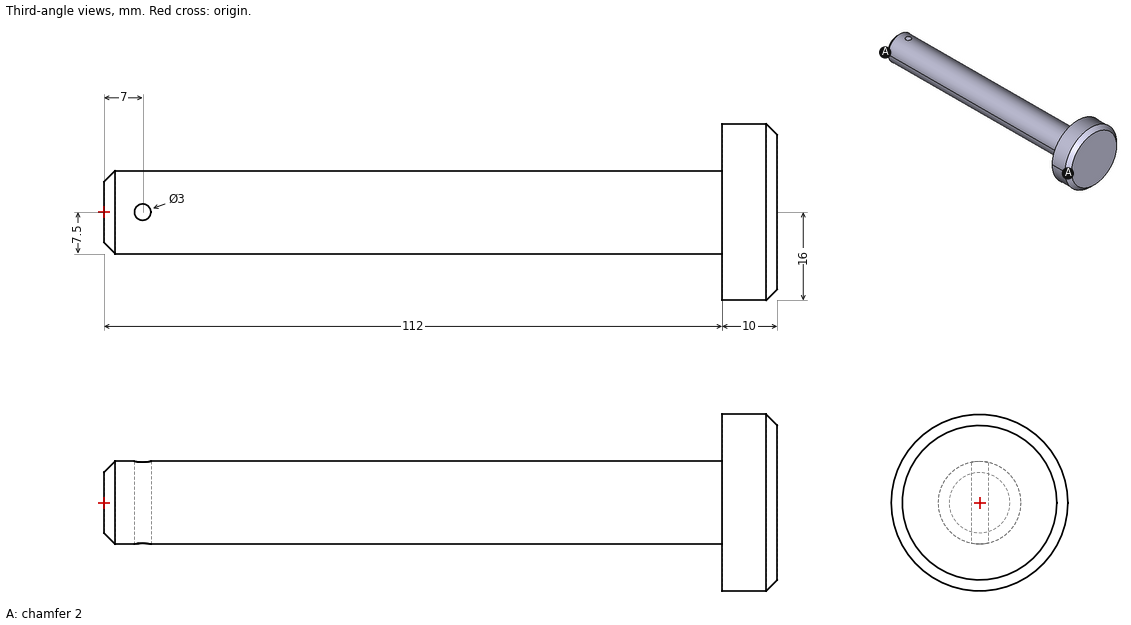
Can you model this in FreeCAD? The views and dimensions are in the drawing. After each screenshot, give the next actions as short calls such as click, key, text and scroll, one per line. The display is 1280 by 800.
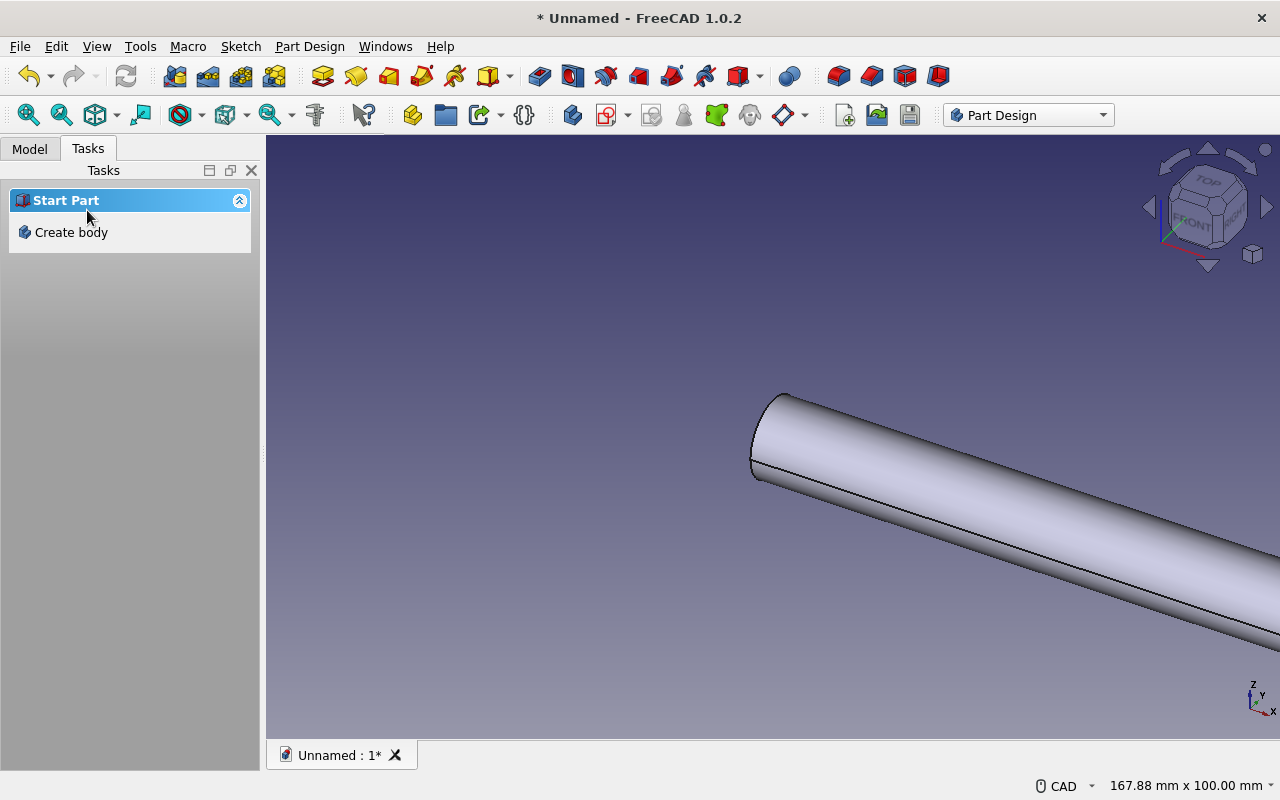
click(29, 116)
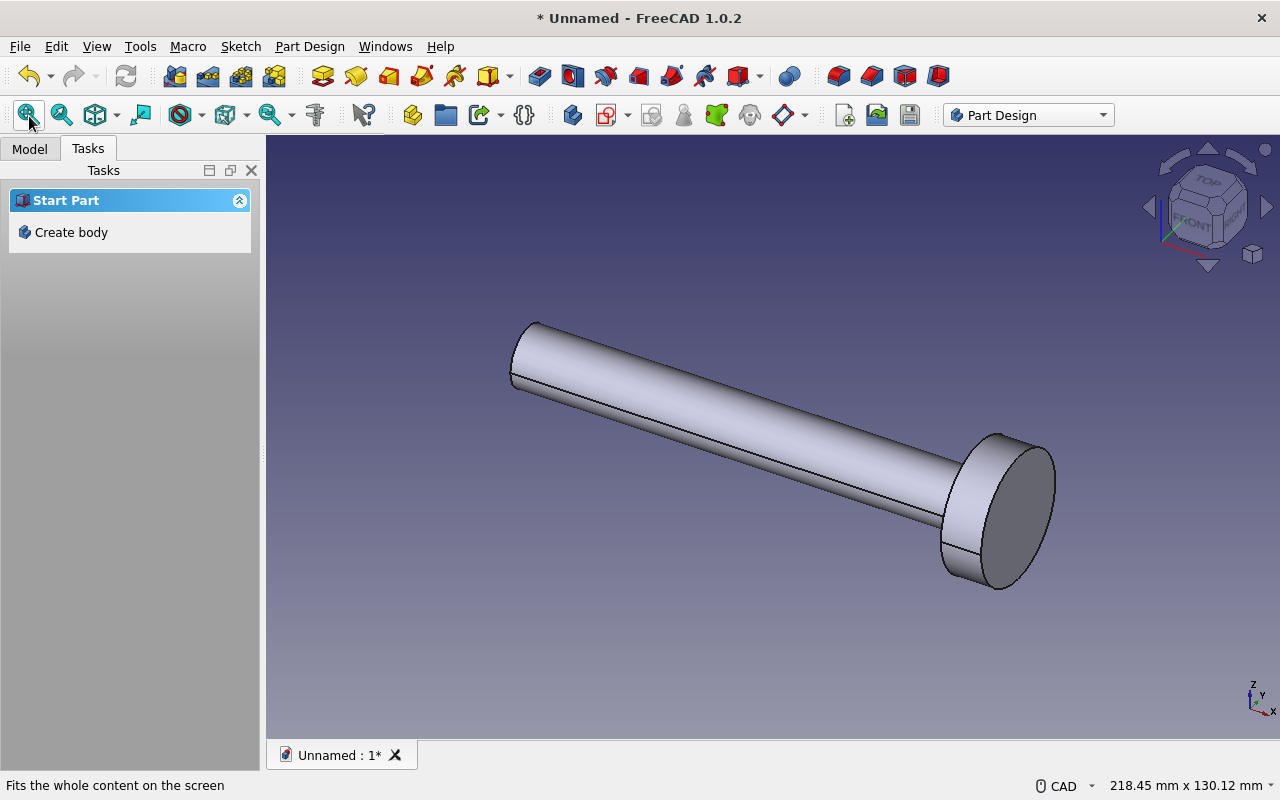
click(606, 116)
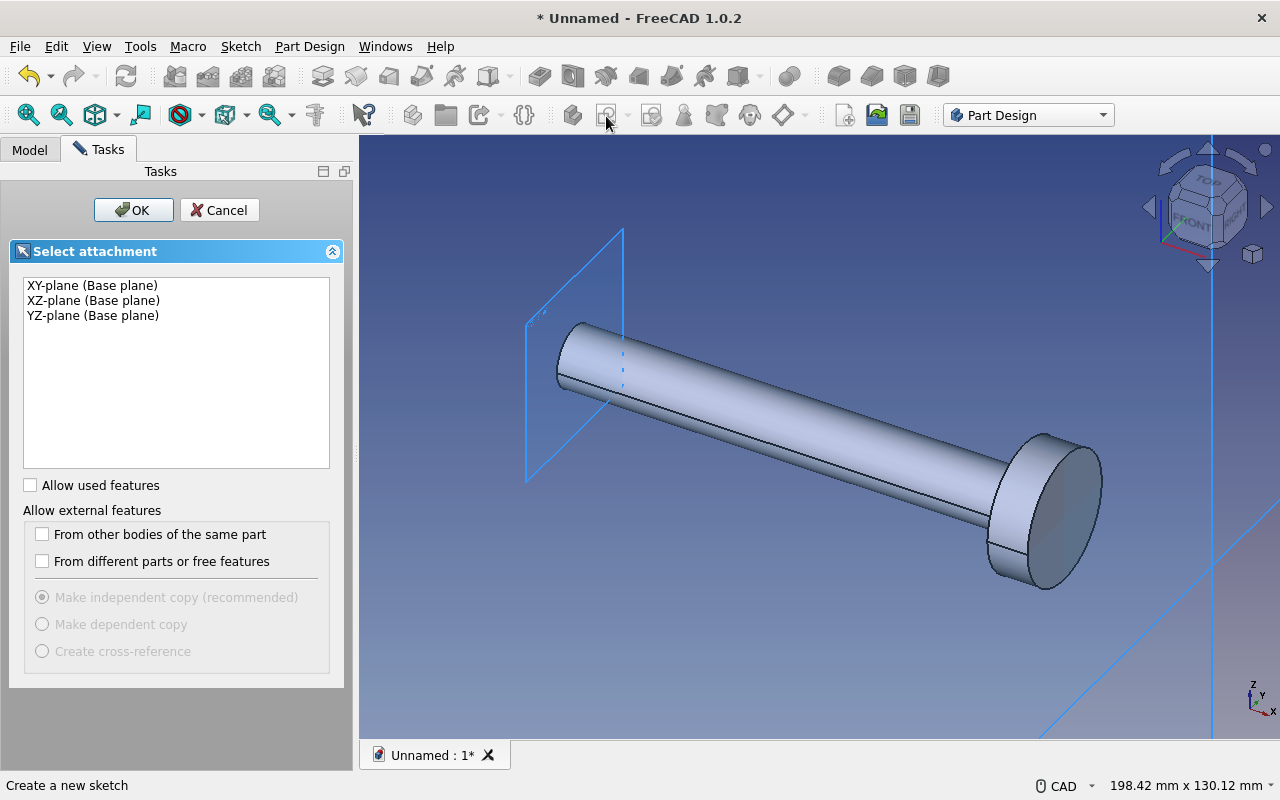
click(84, 286)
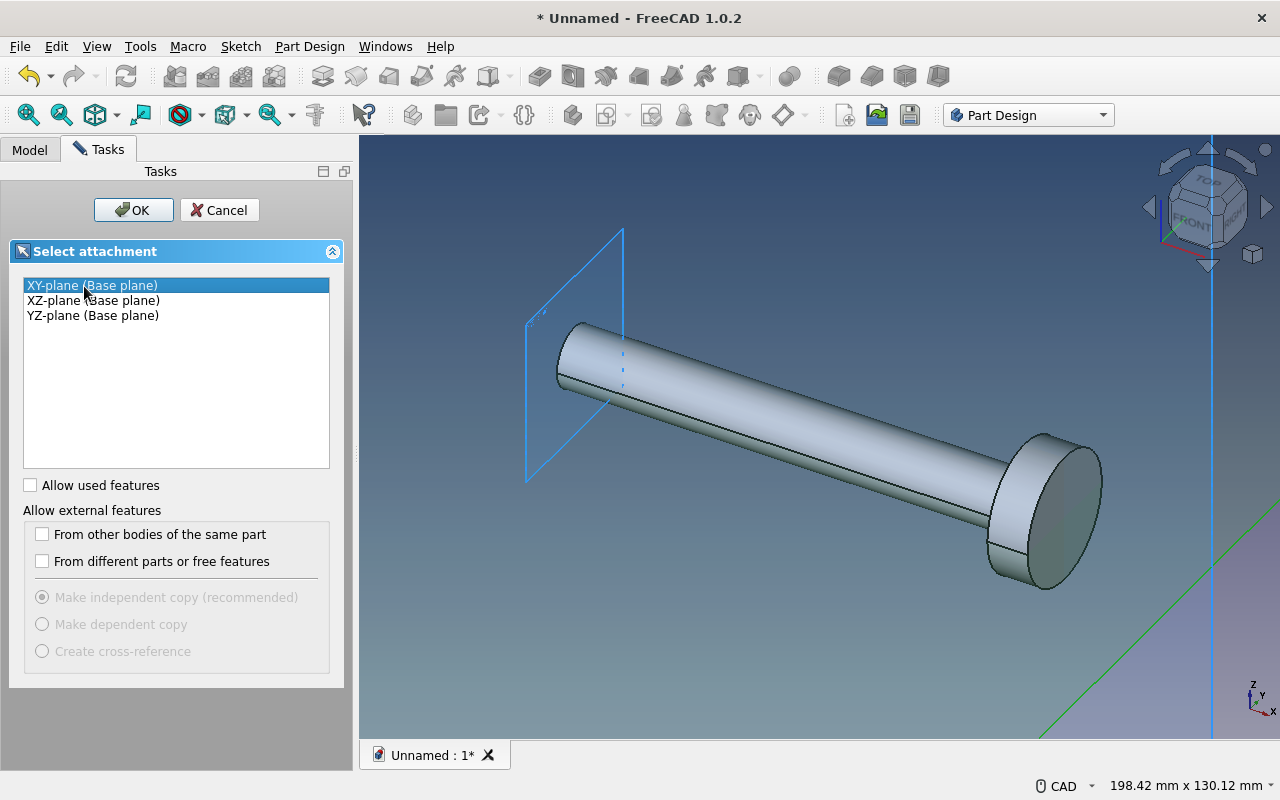
click(134, 210)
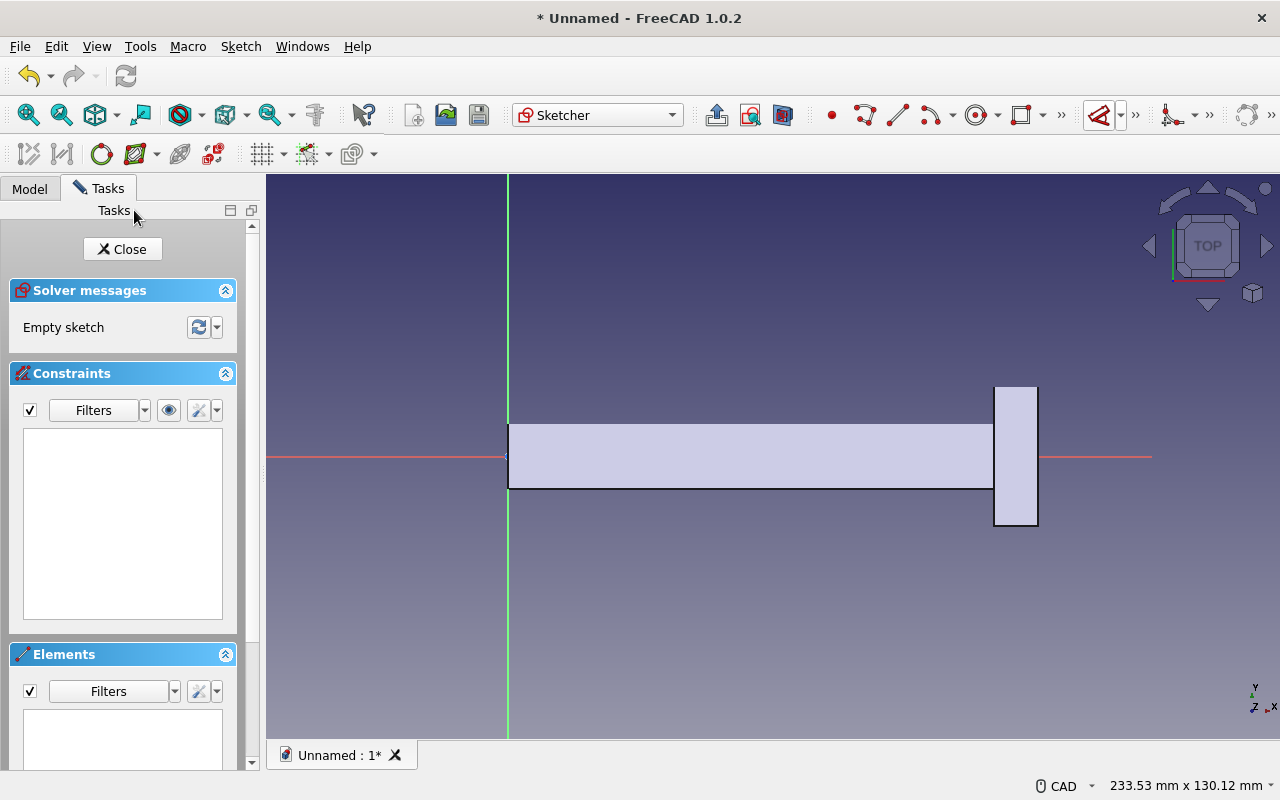
key(q)
key(s)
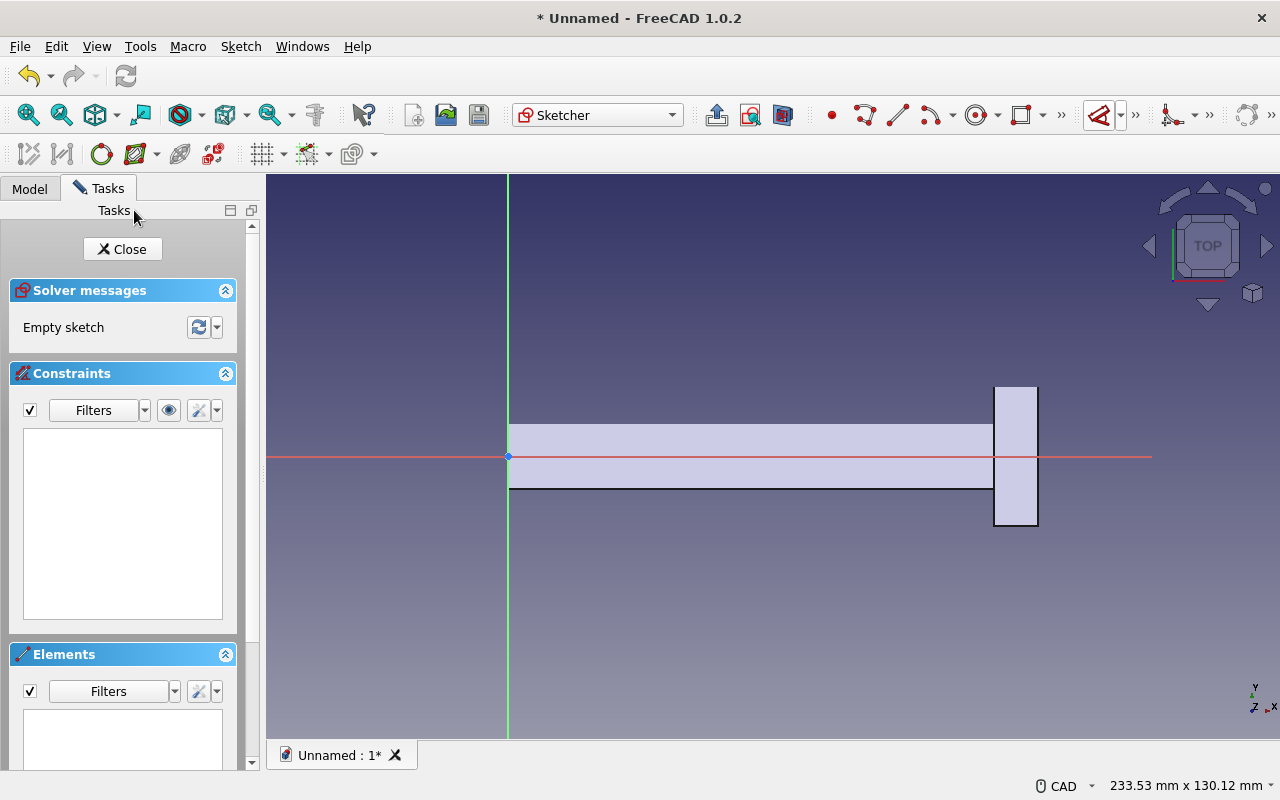
scroll(530, 457, up, 15)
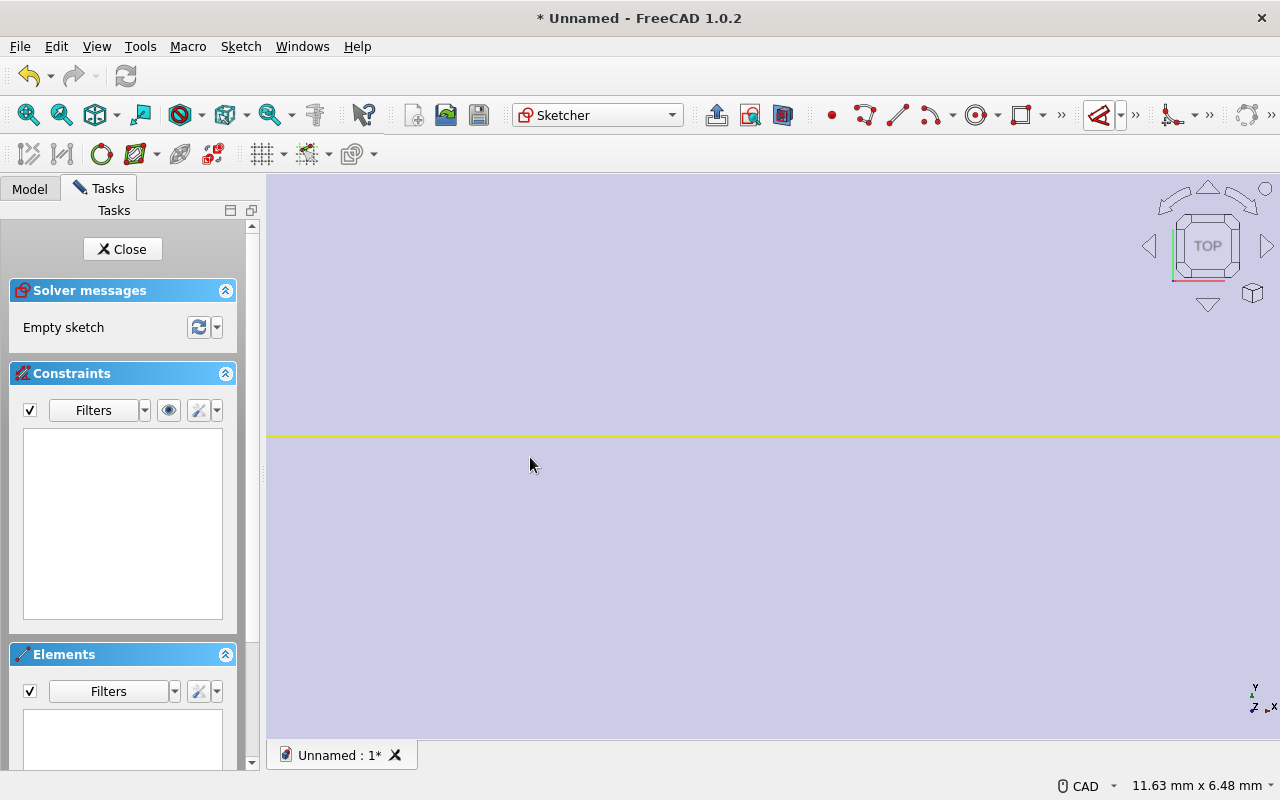
scroll(680, 399, up, 2)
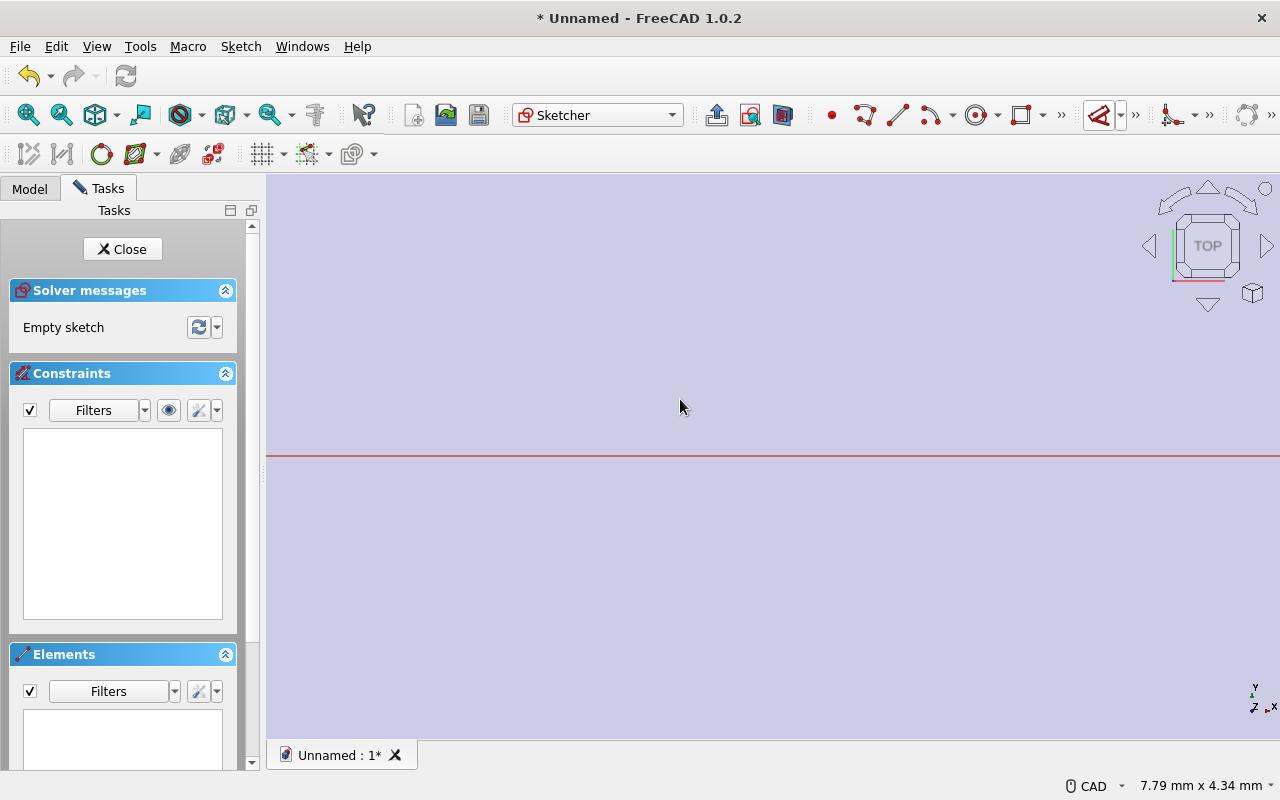
key(g)
key(c)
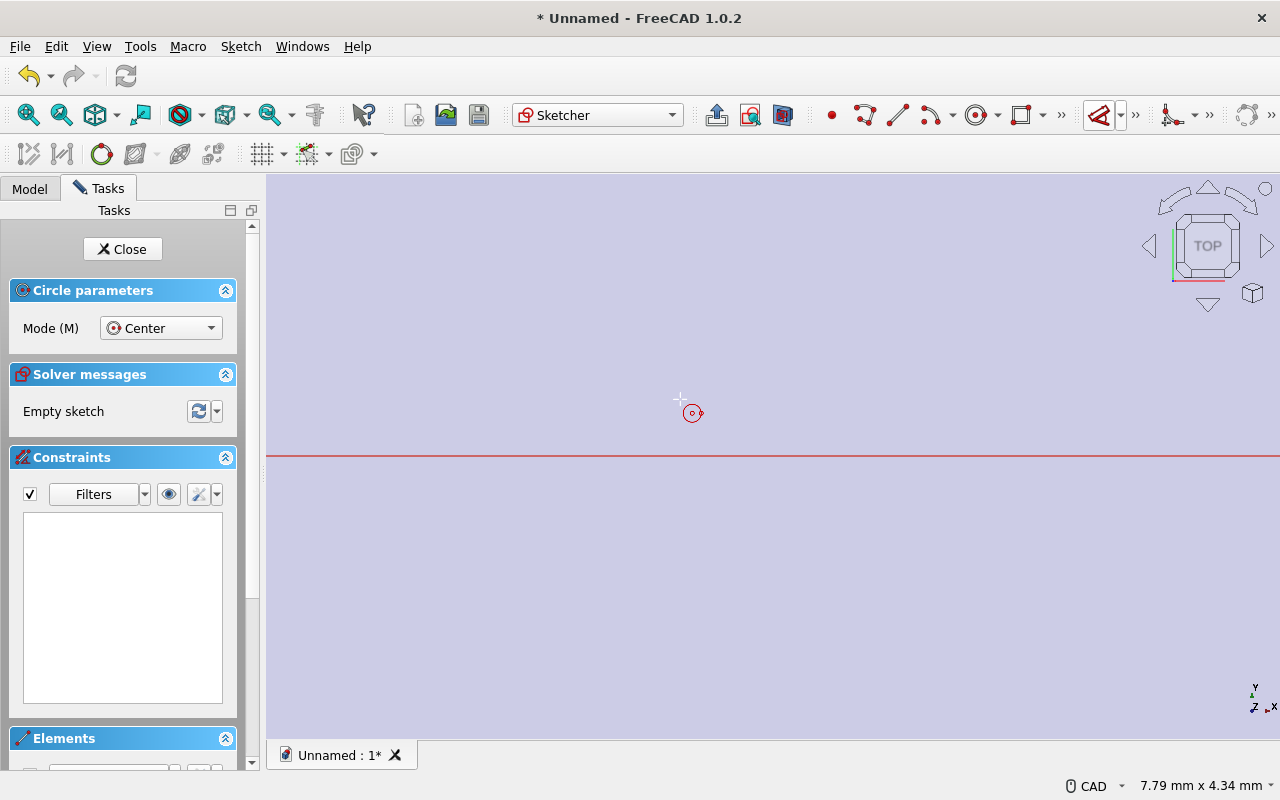
click(704, 456)
move(842, 318)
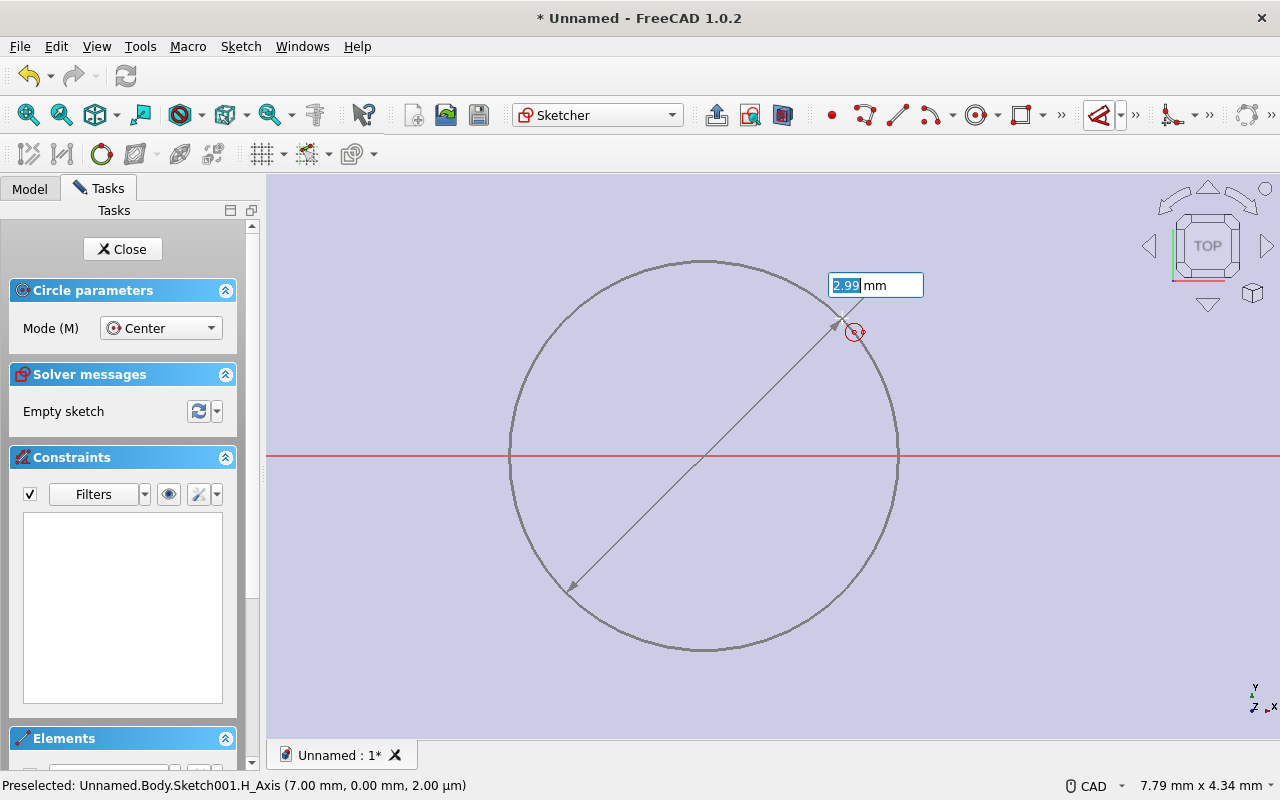
text(3)
key(Return)
key(Escape)